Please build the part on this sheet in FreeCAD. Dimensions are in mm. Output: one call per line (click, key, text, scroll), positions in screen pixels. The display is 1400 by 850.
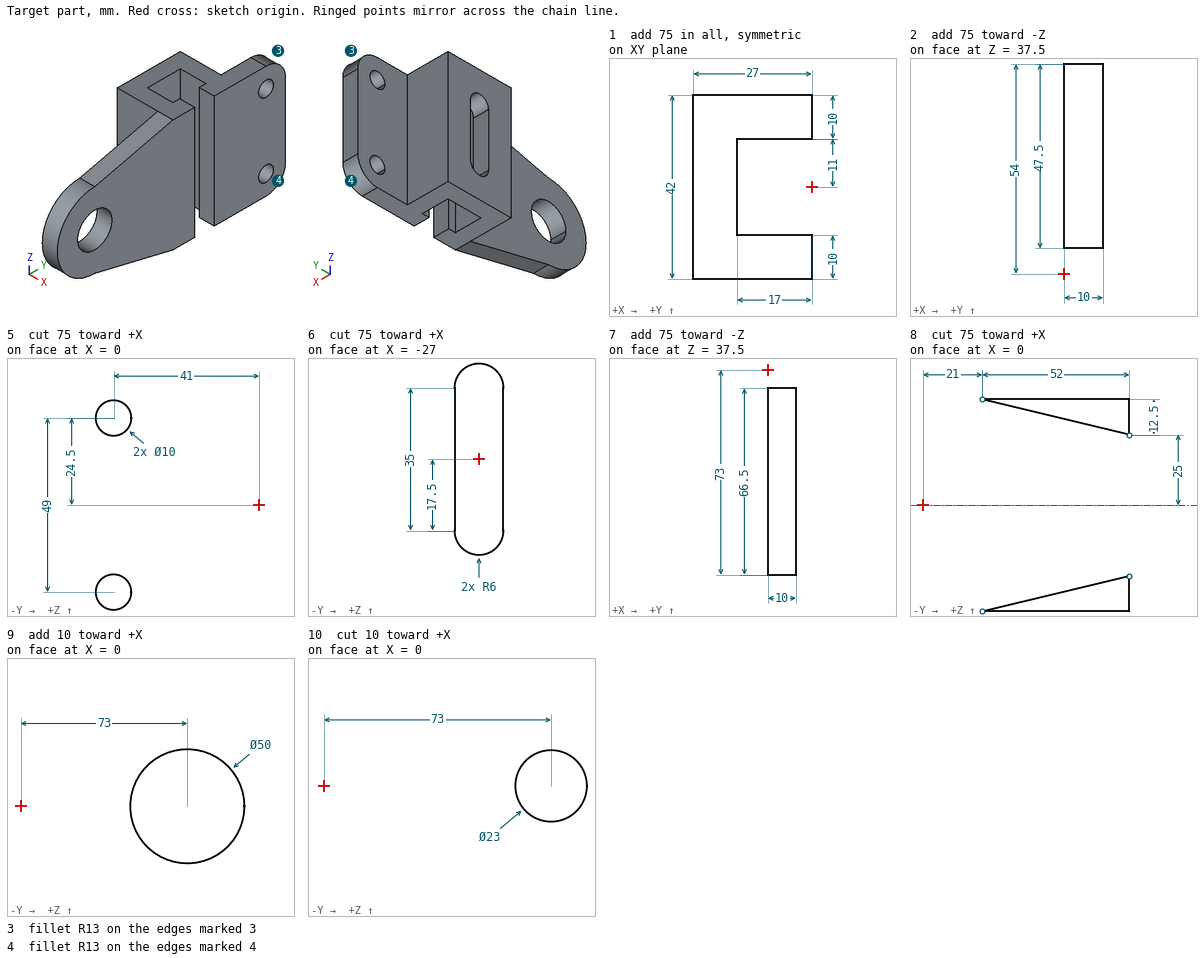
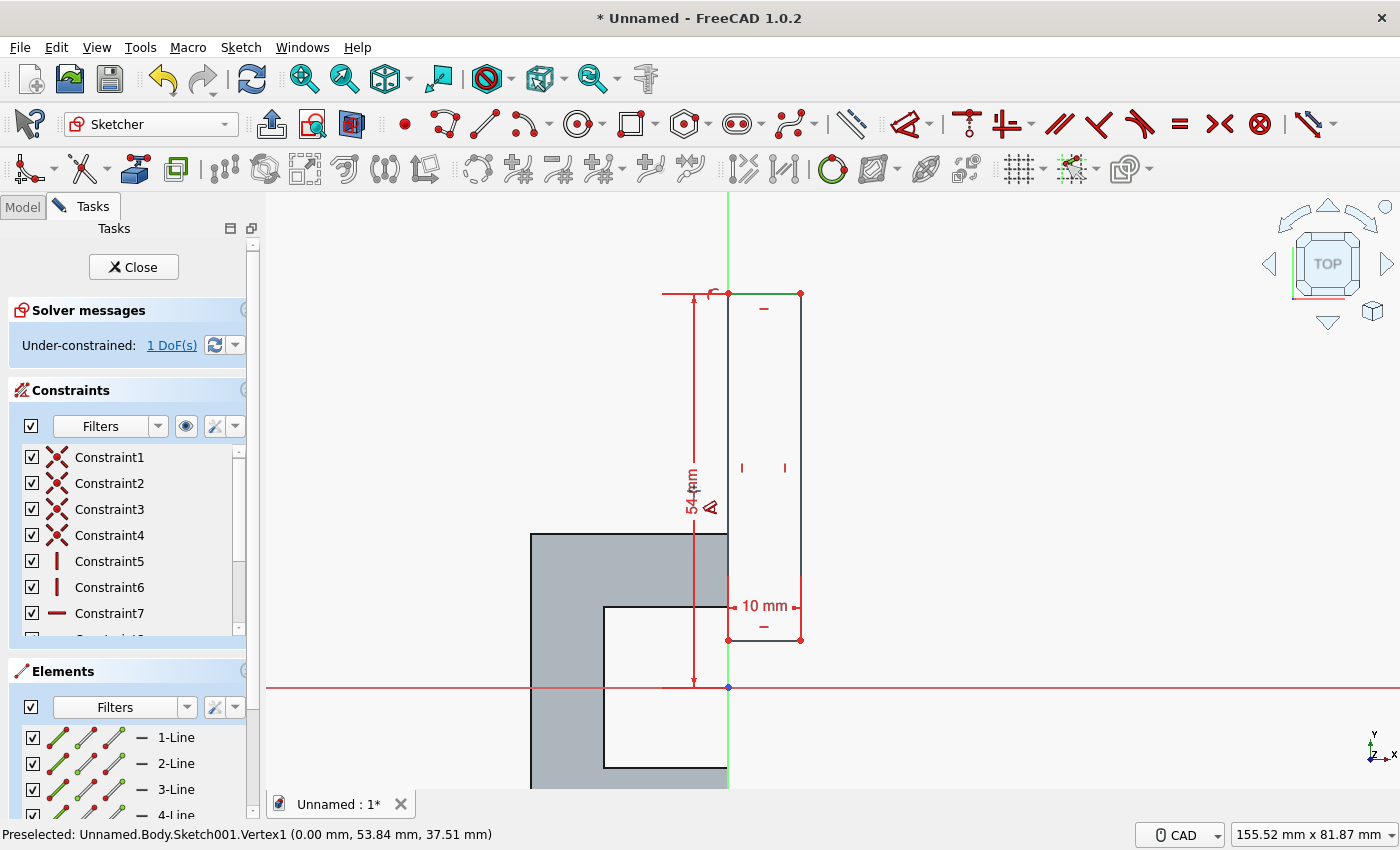
click(728, 398)
click(694, 467)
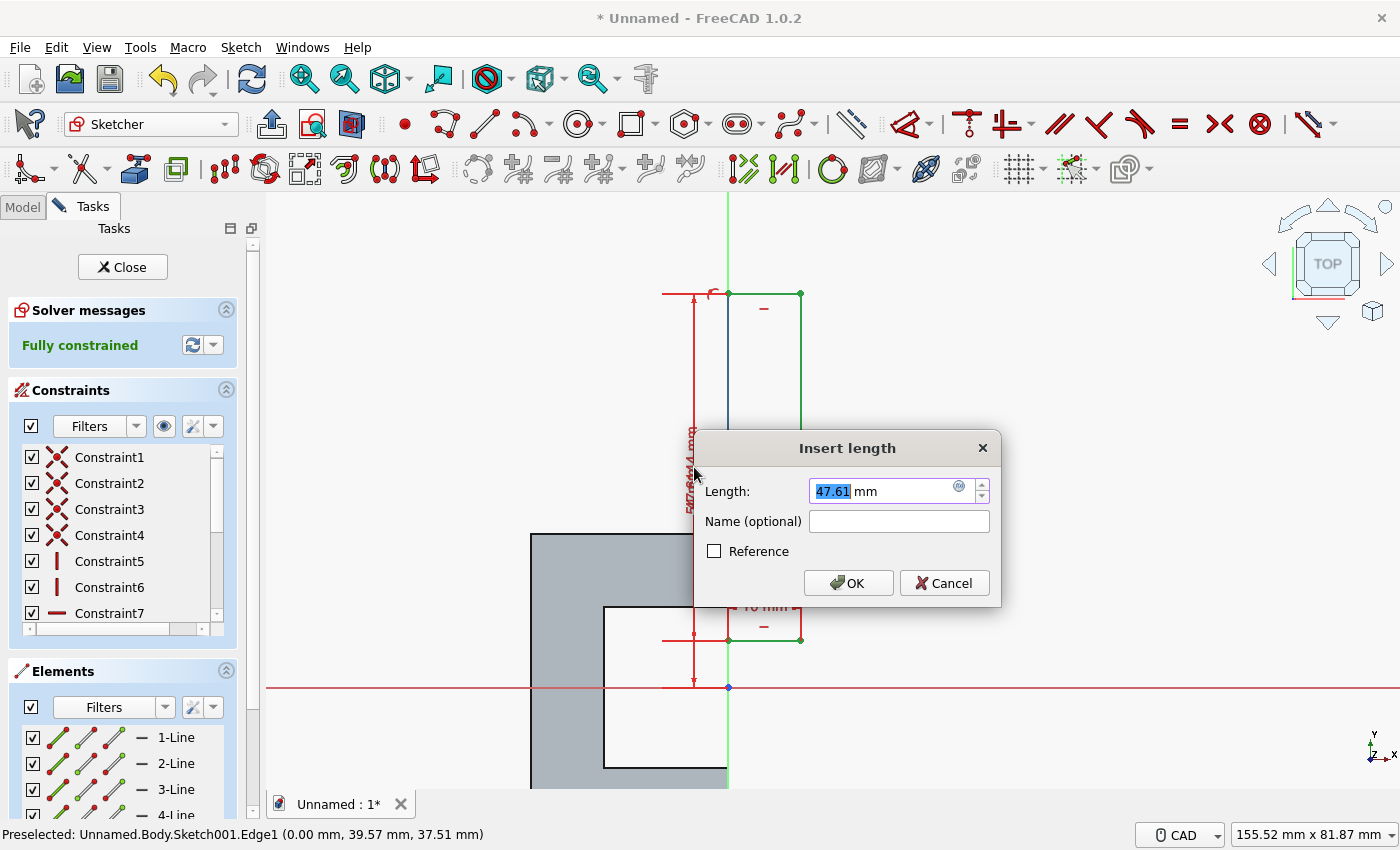
text(47.5)
key(Return)
key(Escape)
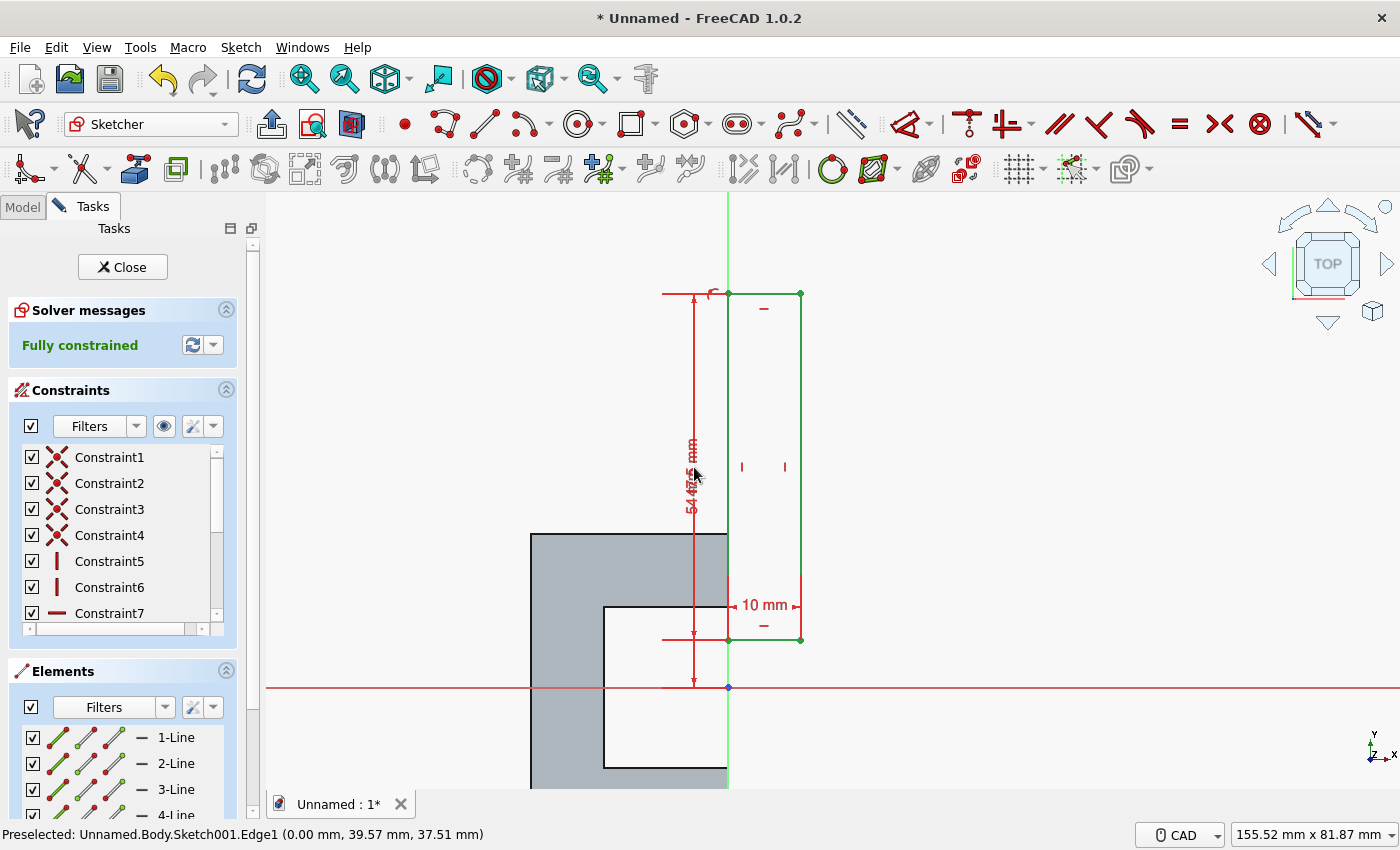
click(123, 267)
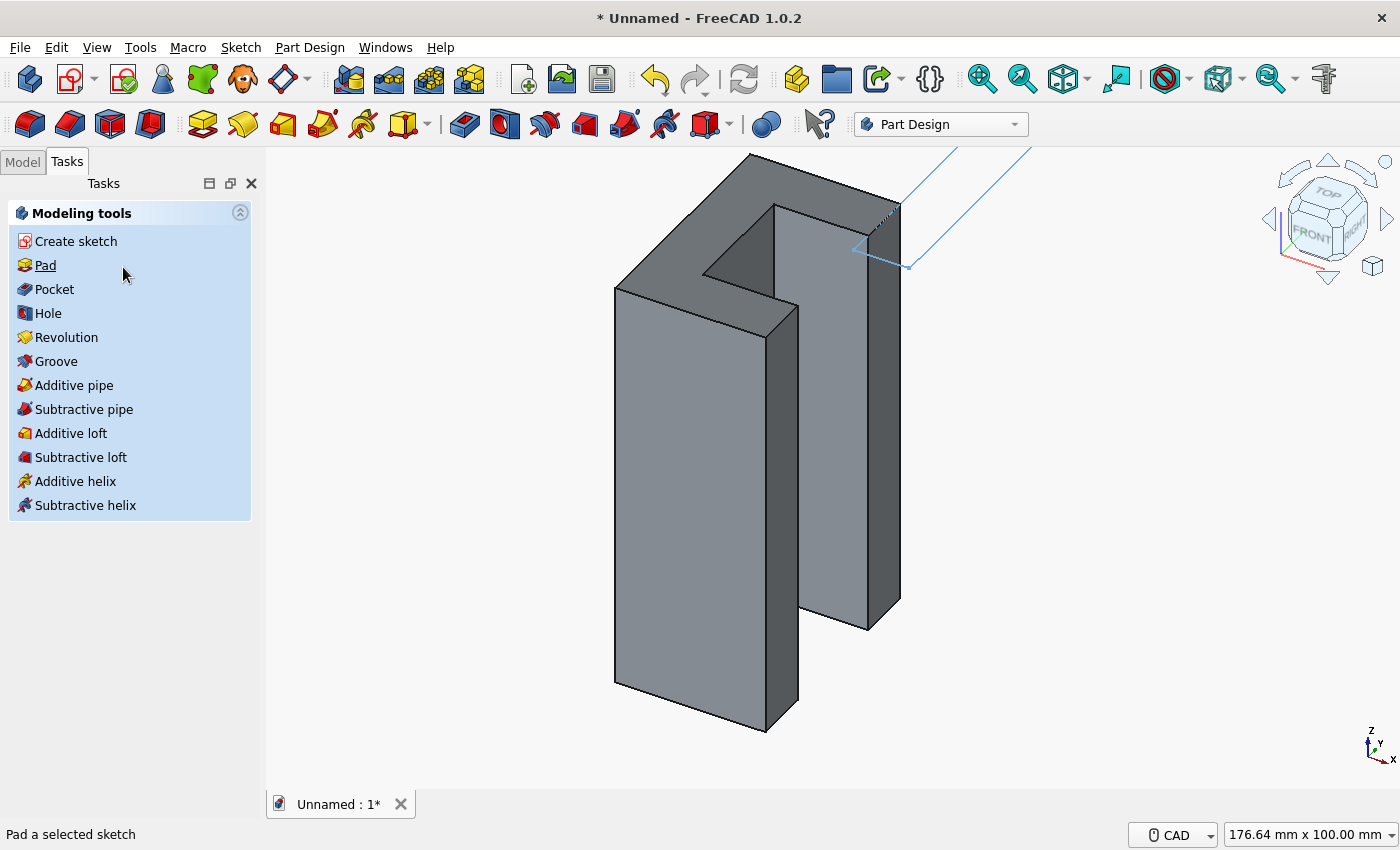
click(204, 124)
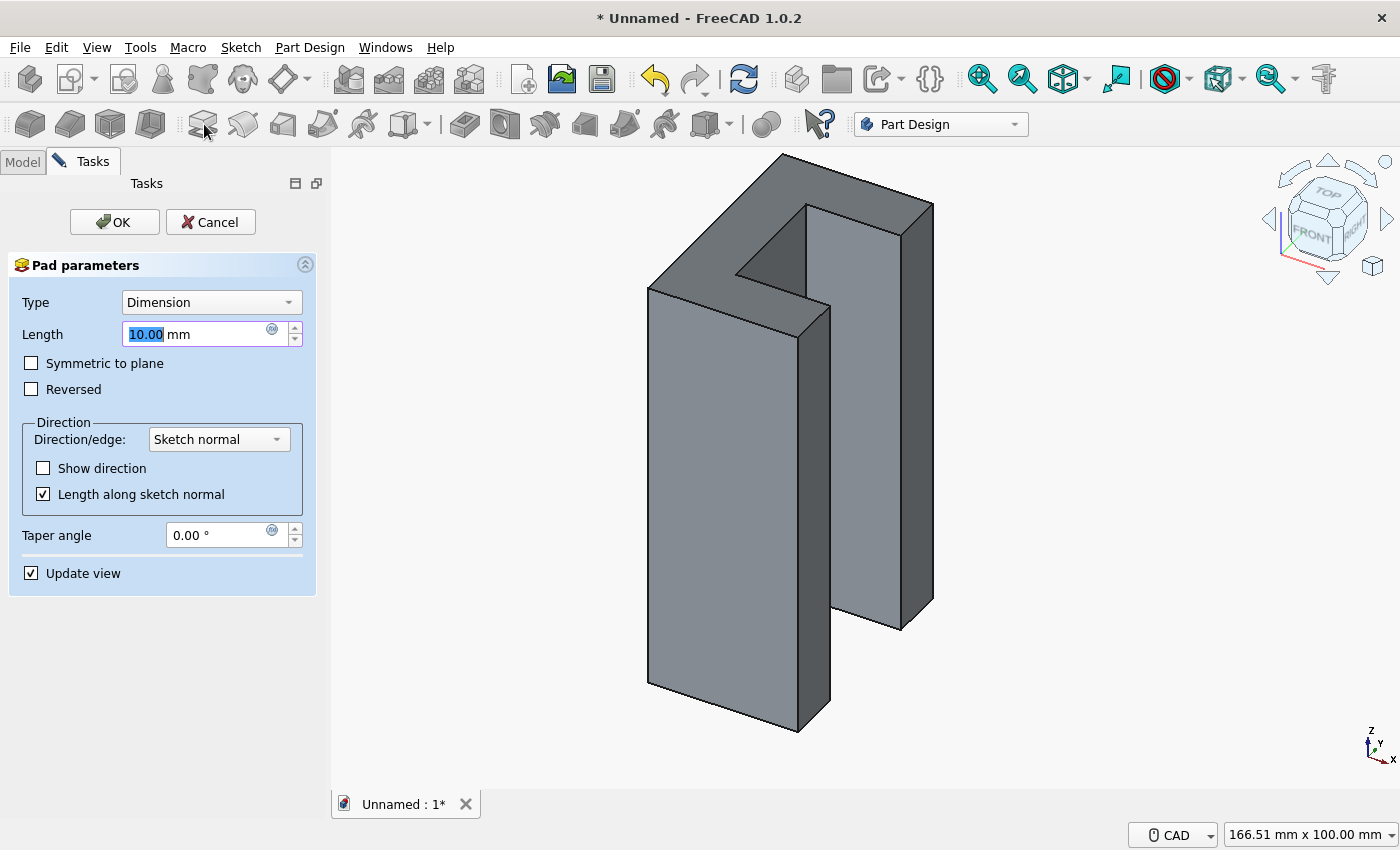
text(75)
key(Tab)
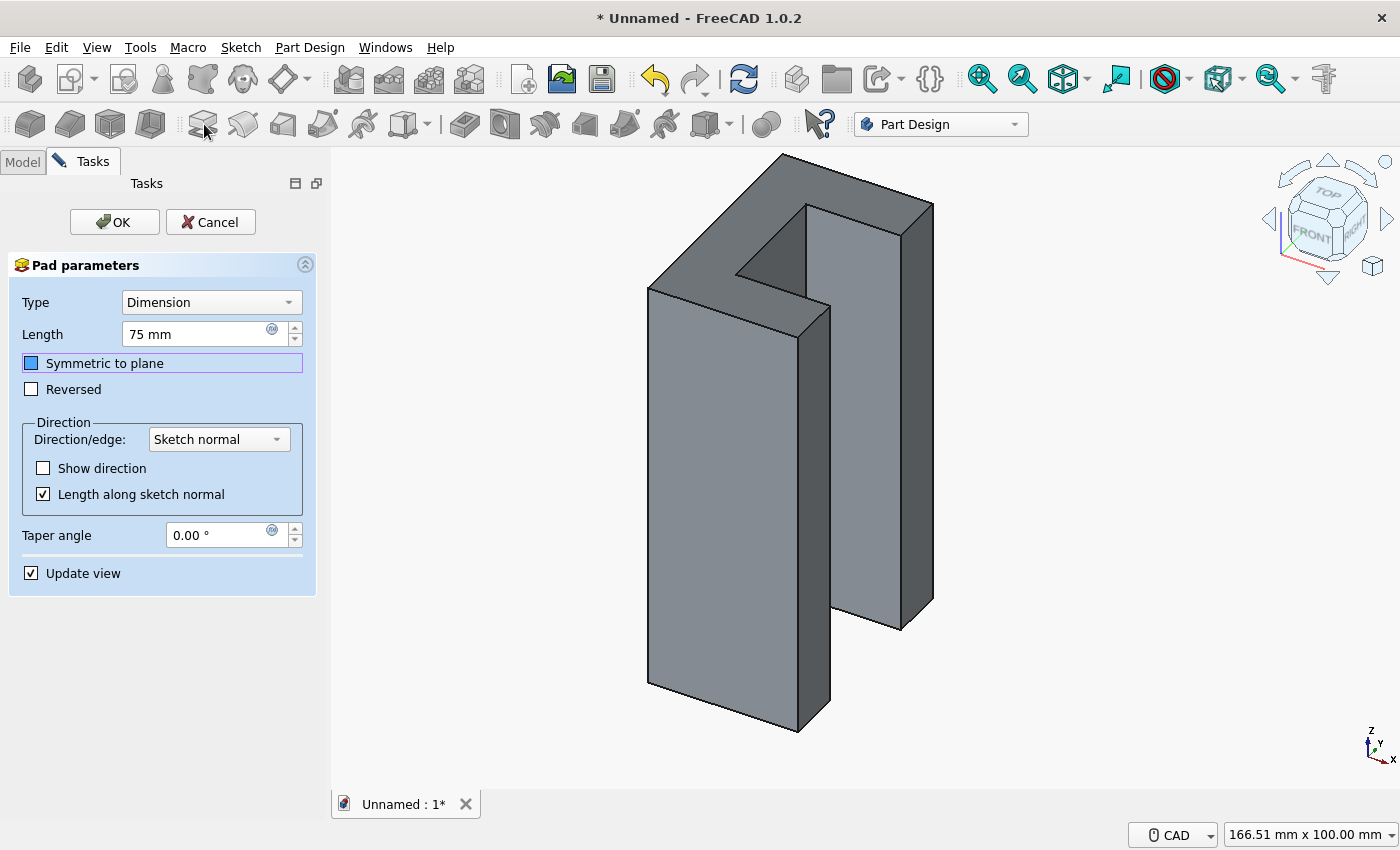
click(30, 389)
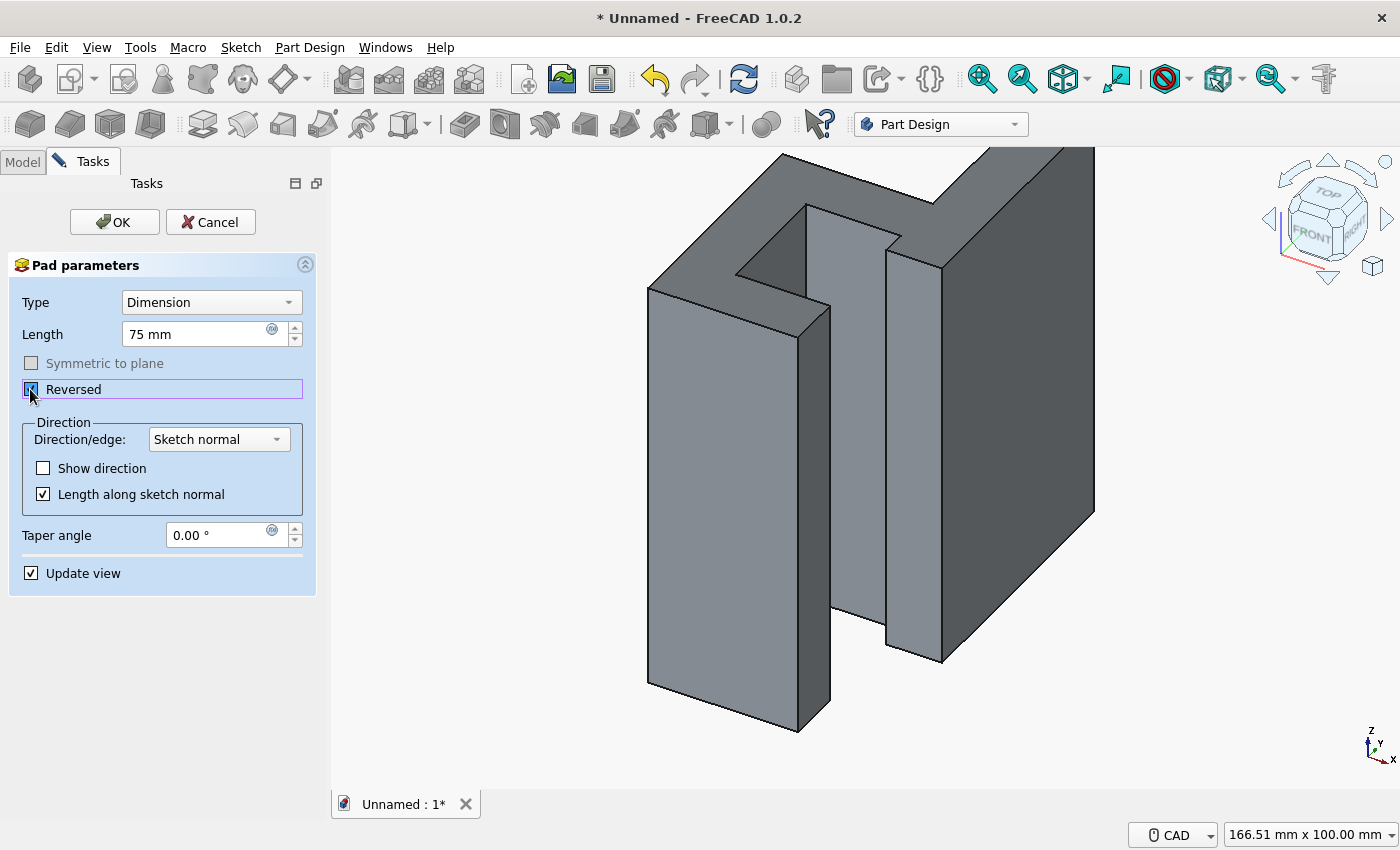
click(115, 222)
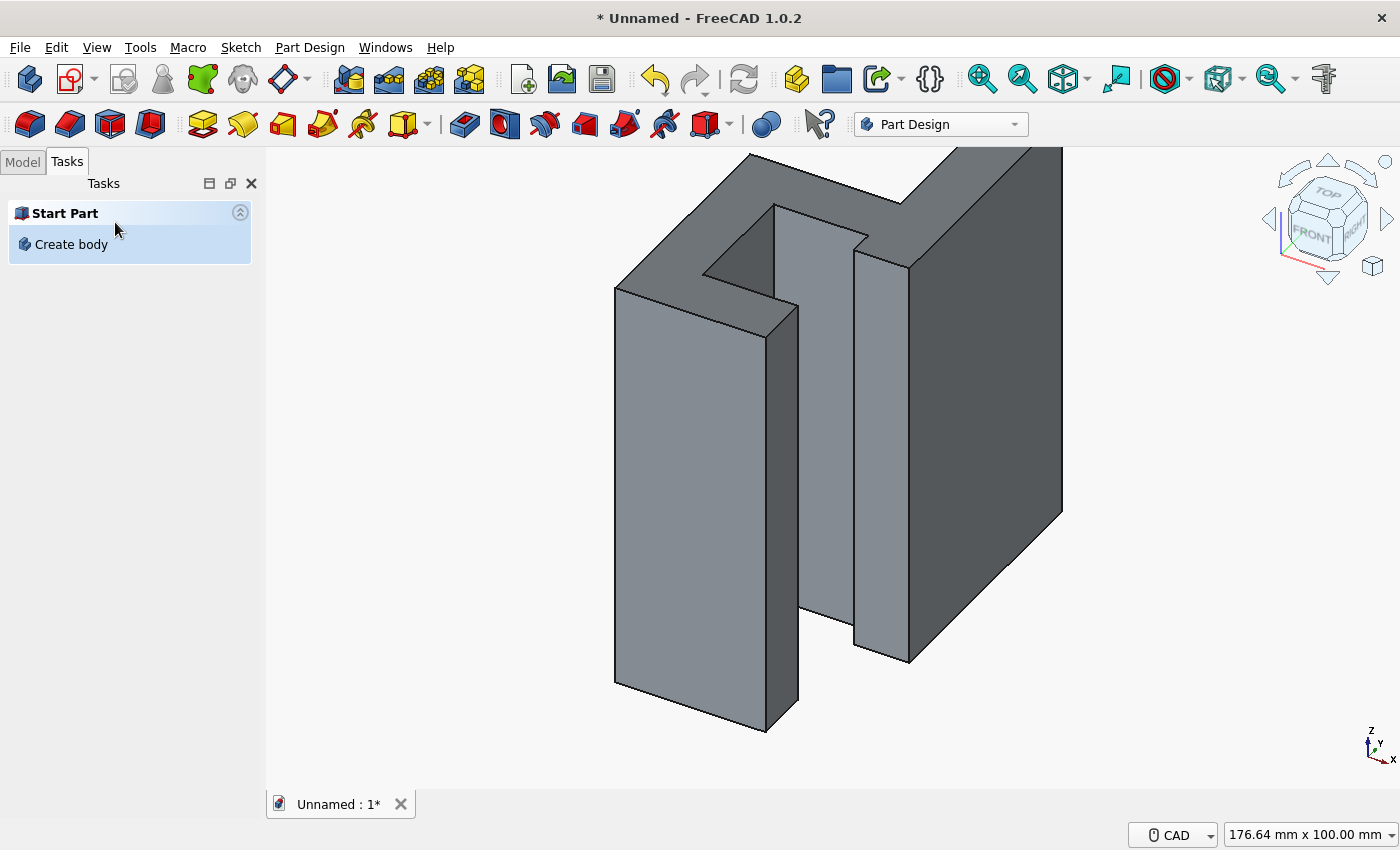
key(v)
key(f)